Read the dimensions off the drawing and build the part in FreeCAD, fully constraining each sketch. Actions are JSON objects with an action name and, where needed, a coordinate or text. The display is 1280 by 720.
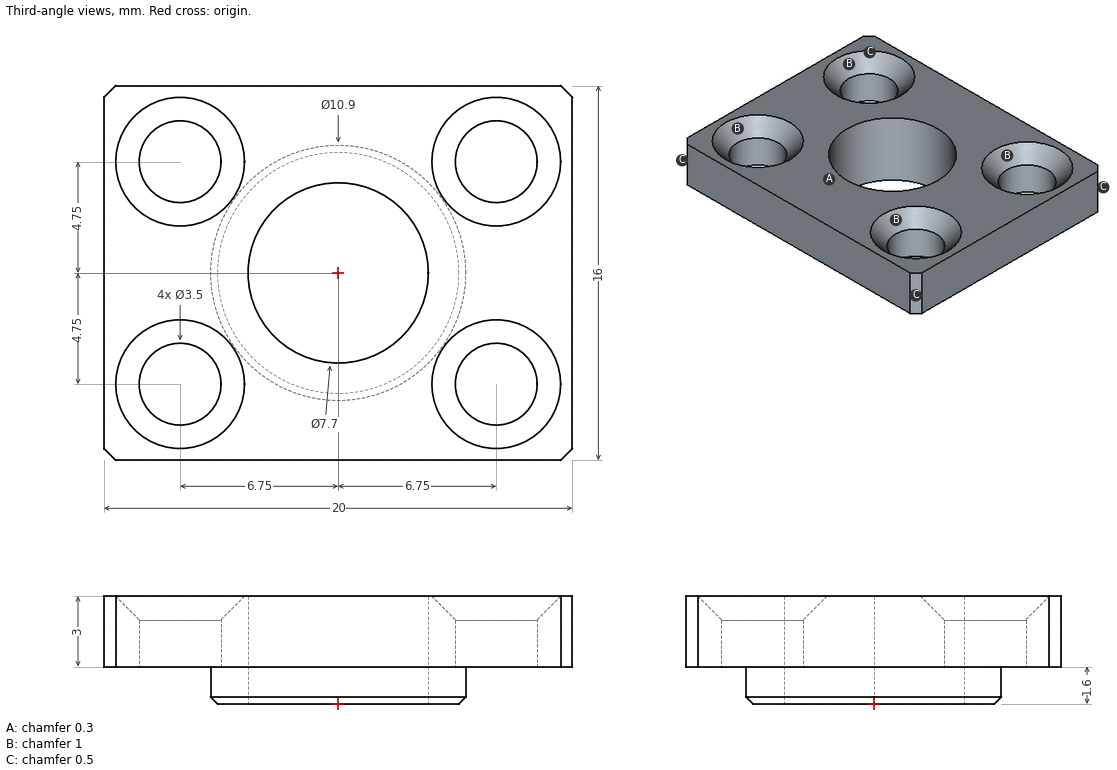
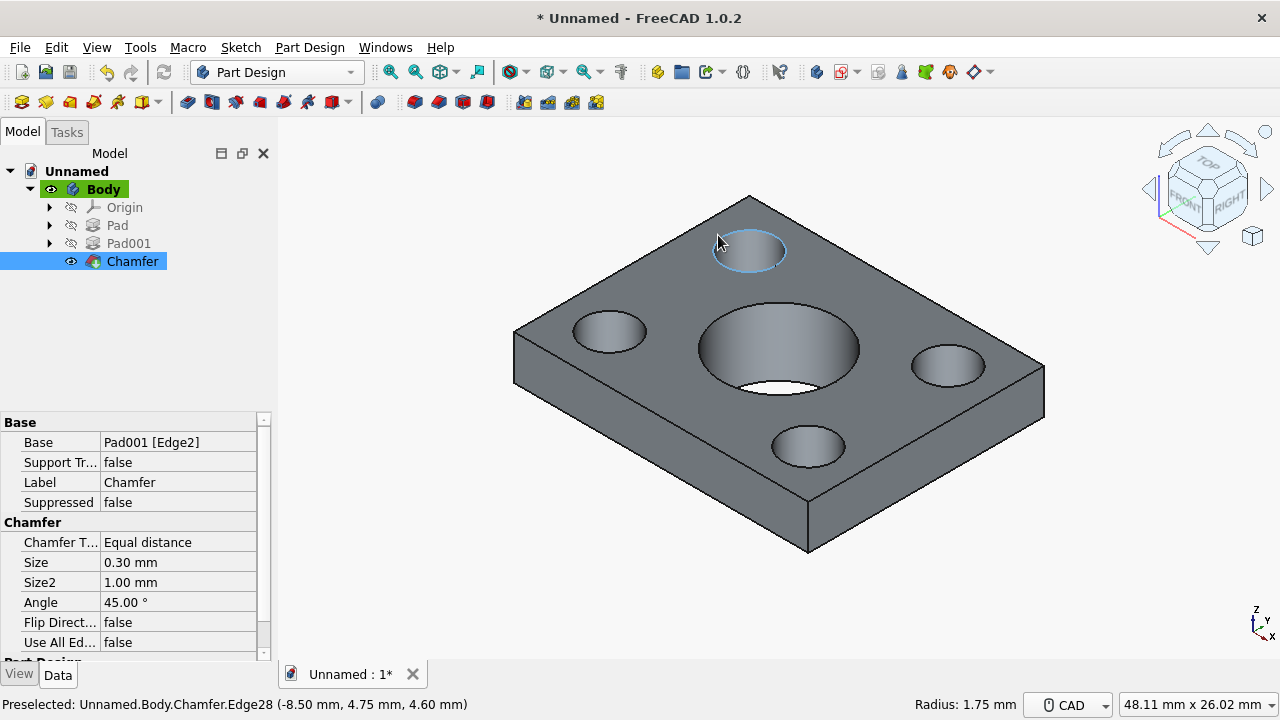
{"action": "left_click", "coordinate": [584, 316], "text": "ctrl"}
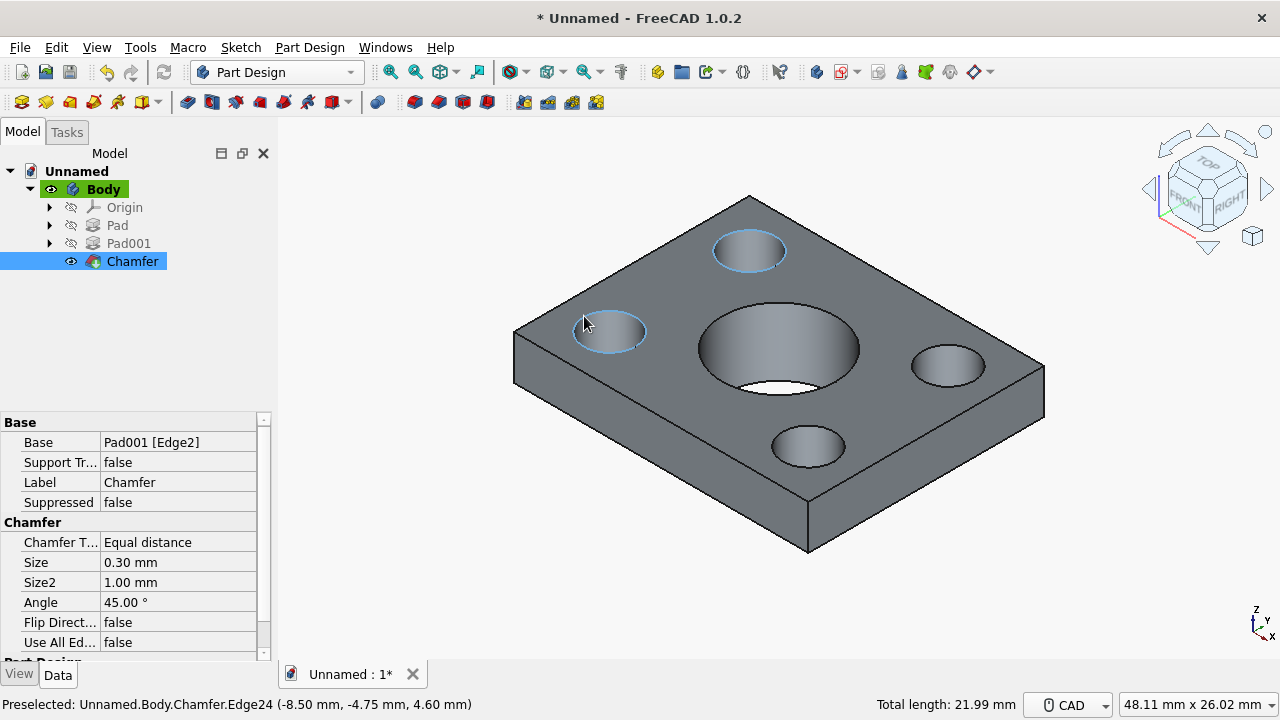
{"action": "left_click", "coordinate": [783, 431], "text": "ctrl"}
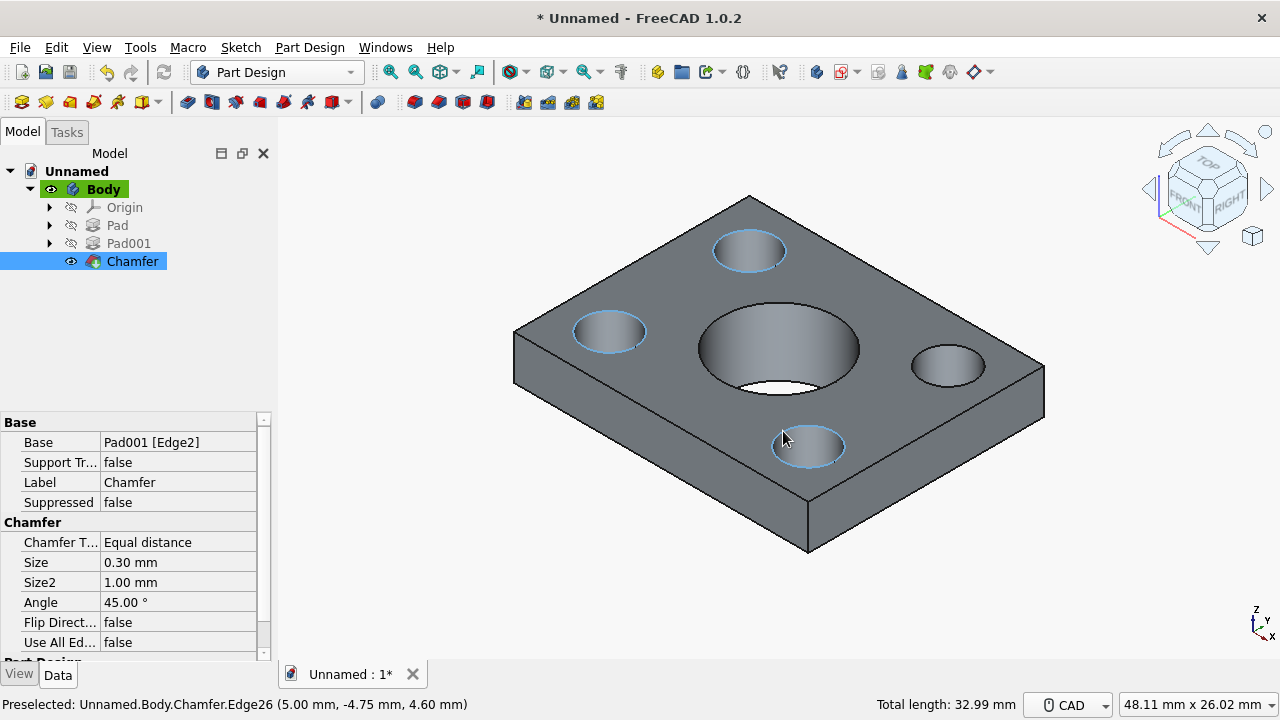
{"action": "left_click", "coordinate": [923, 350], "text": "ctrl"}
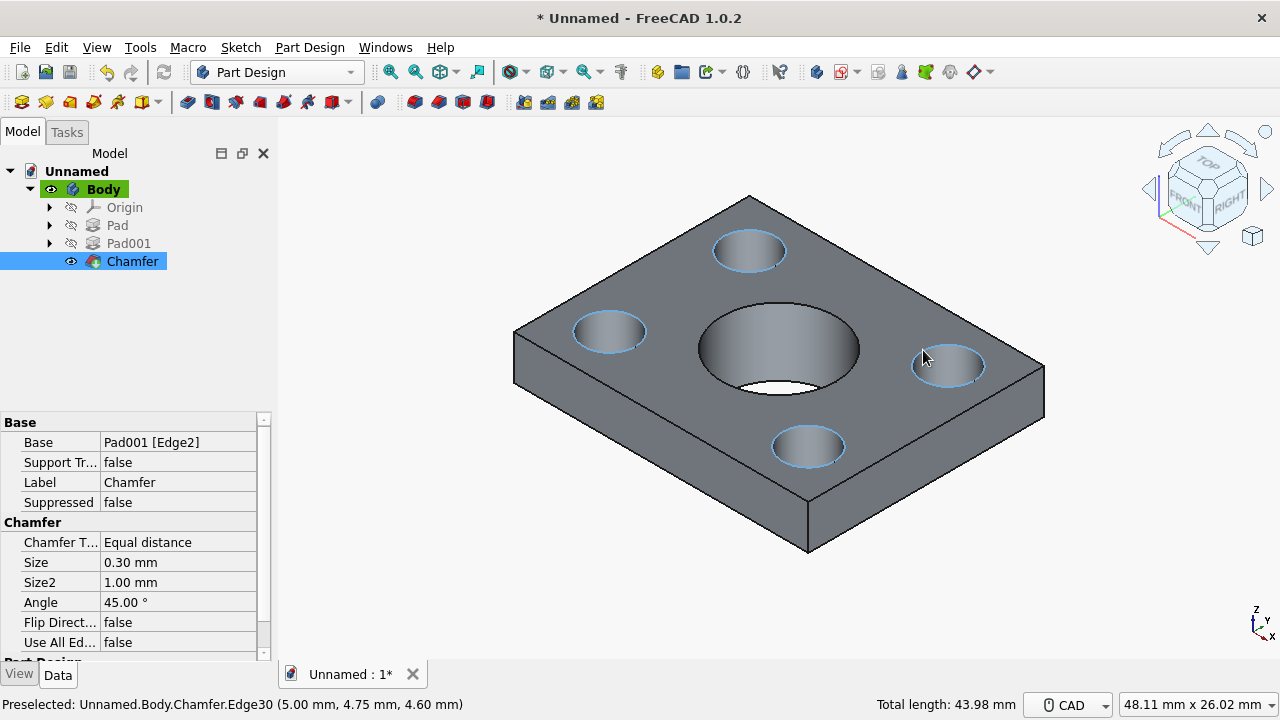
{"action": "left_click", "coordinate": [440, 102]}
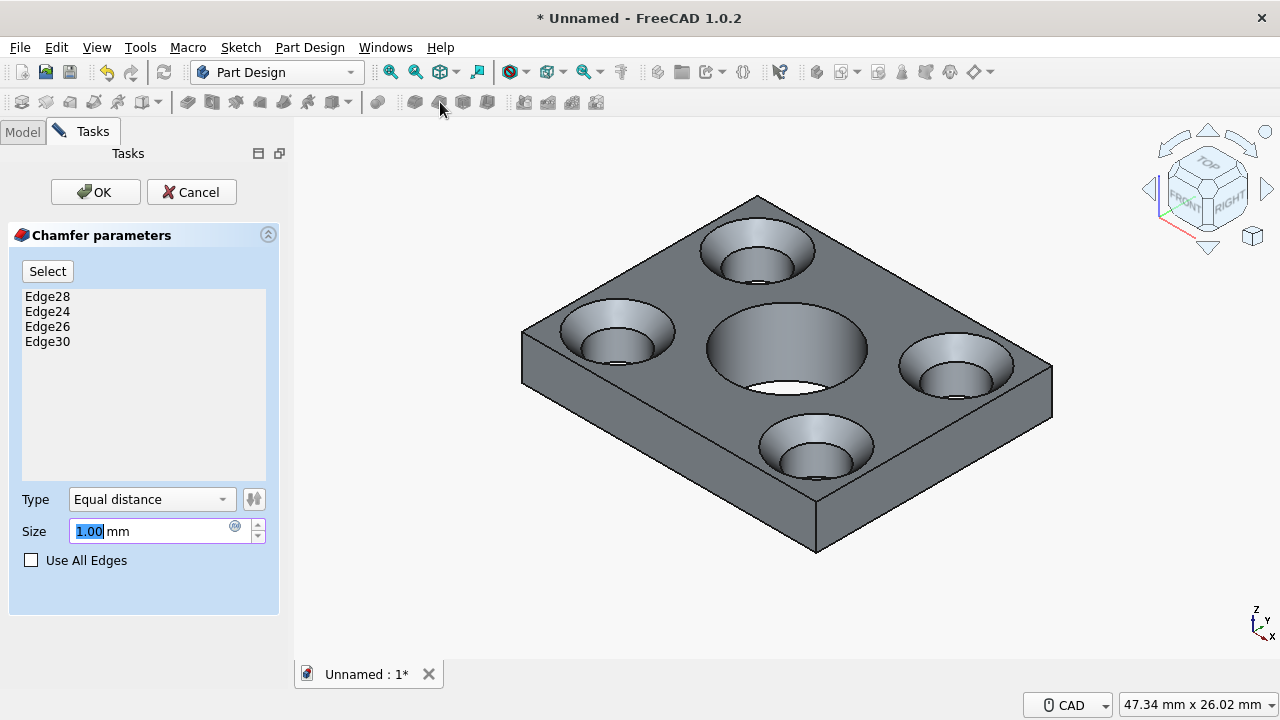
{"action": "type", "text": "1"}
{"action": "key", "text": "Tab"}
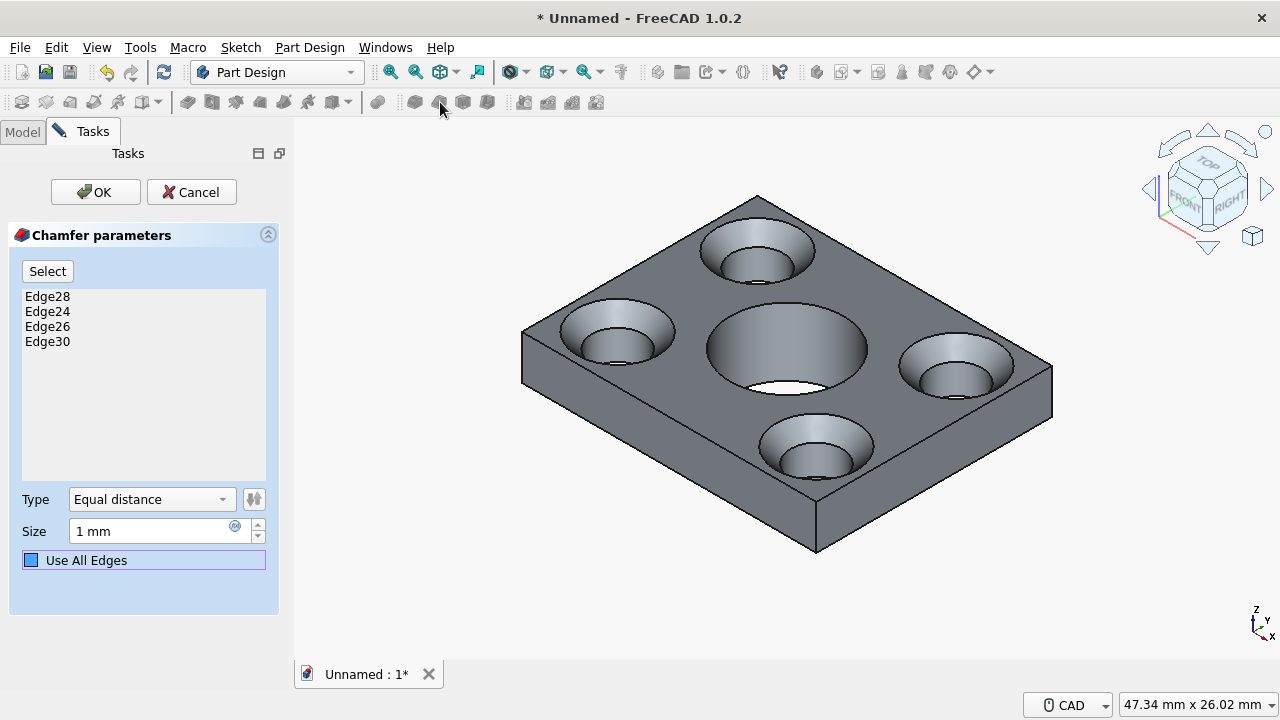
{"action": "left_click", "coordinate": [96, 192]}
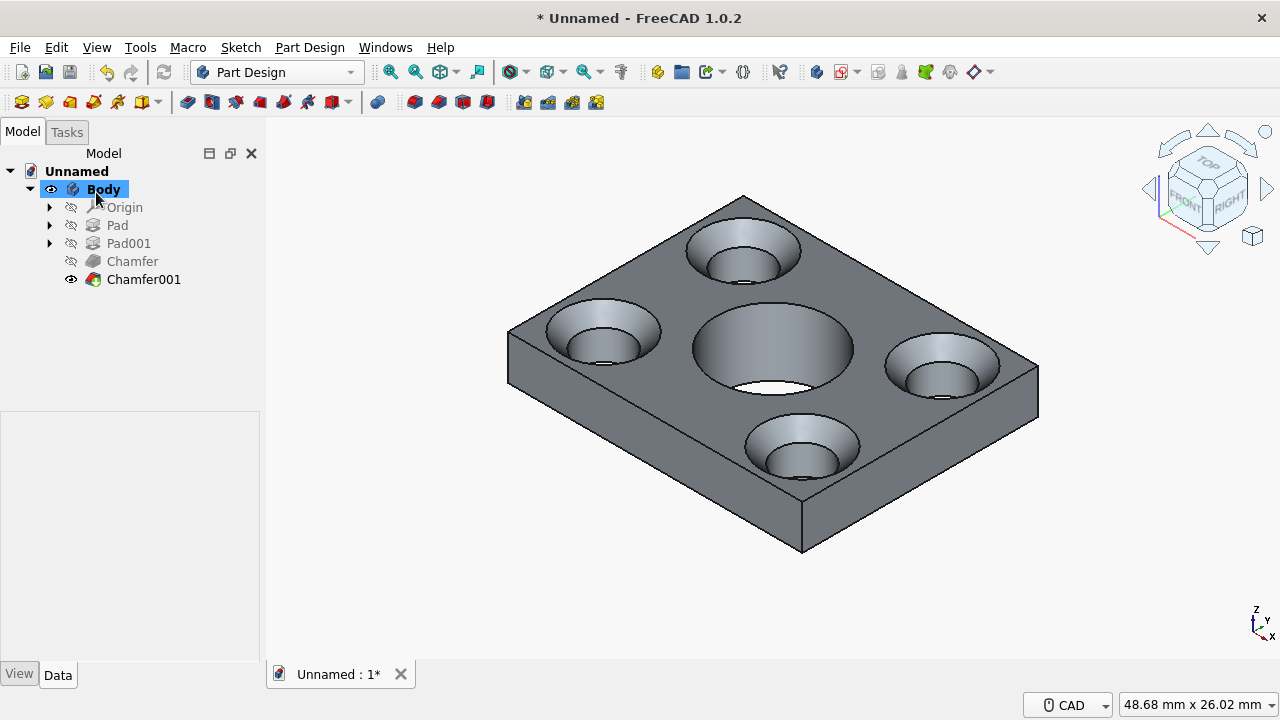
{"action": "left_click", "coordinate": [802, 526]}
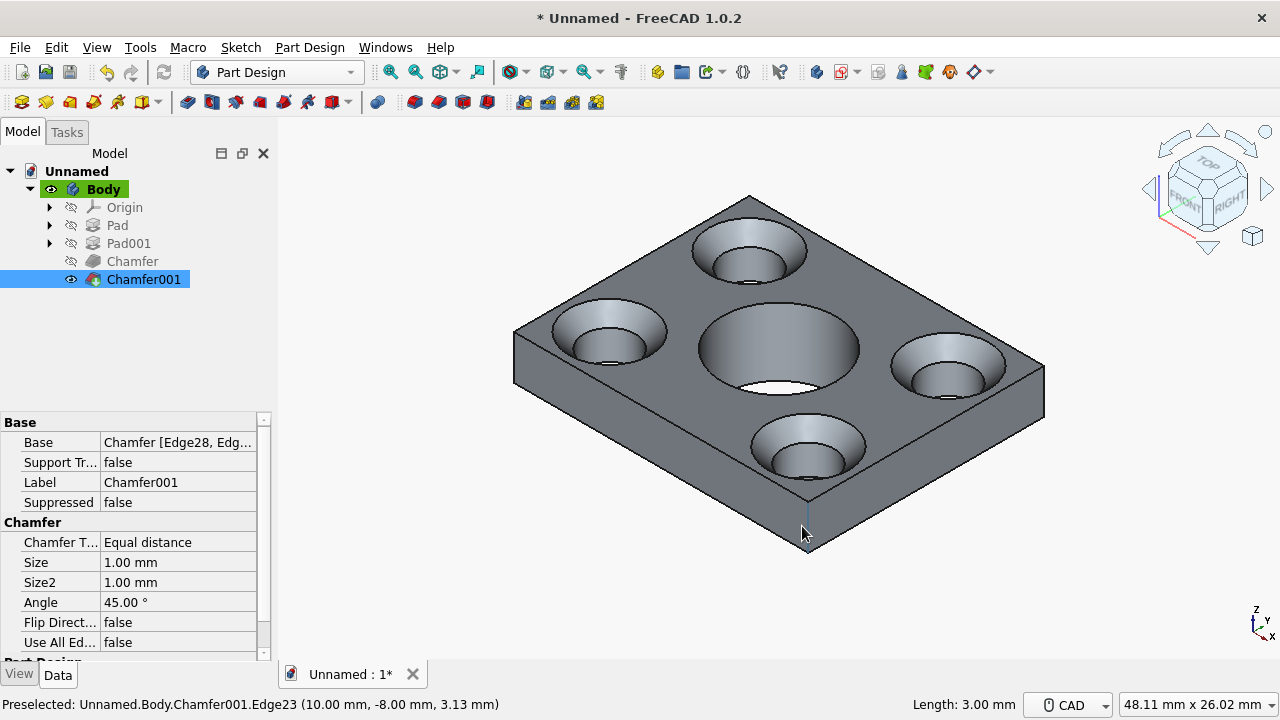
{"action": "key", "text": "2"}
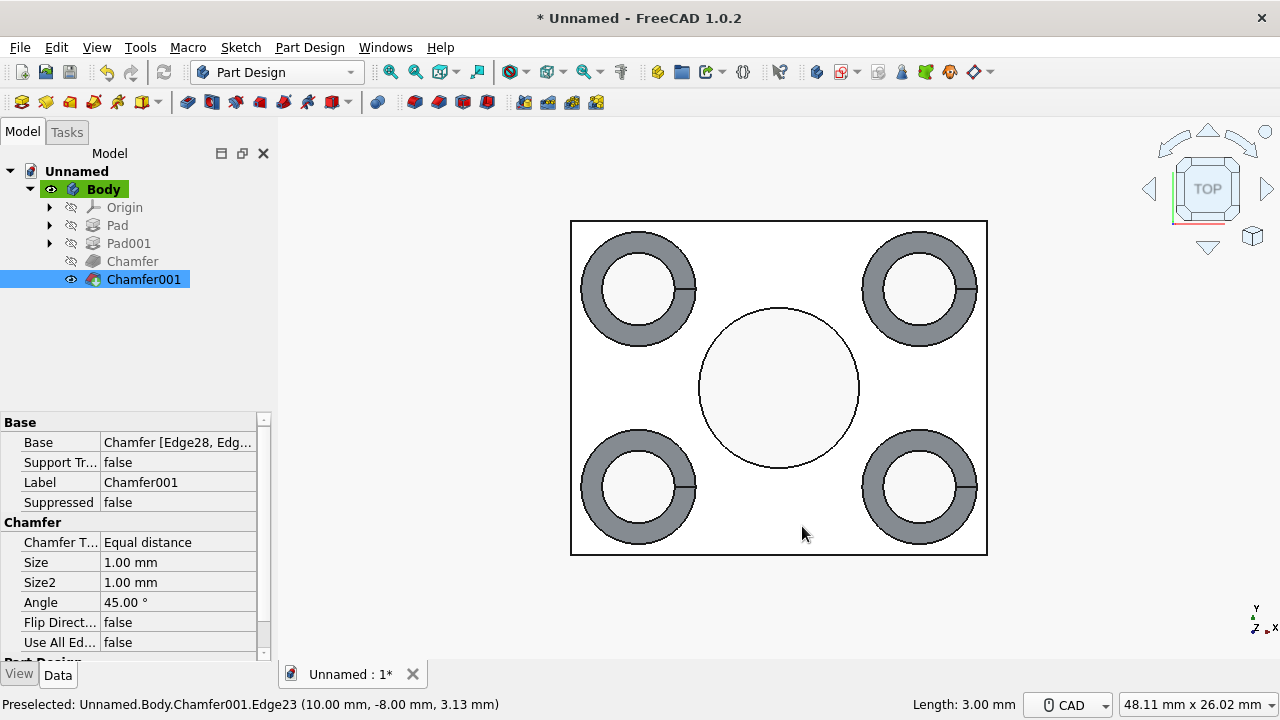
{"action": "key", "text": "0"}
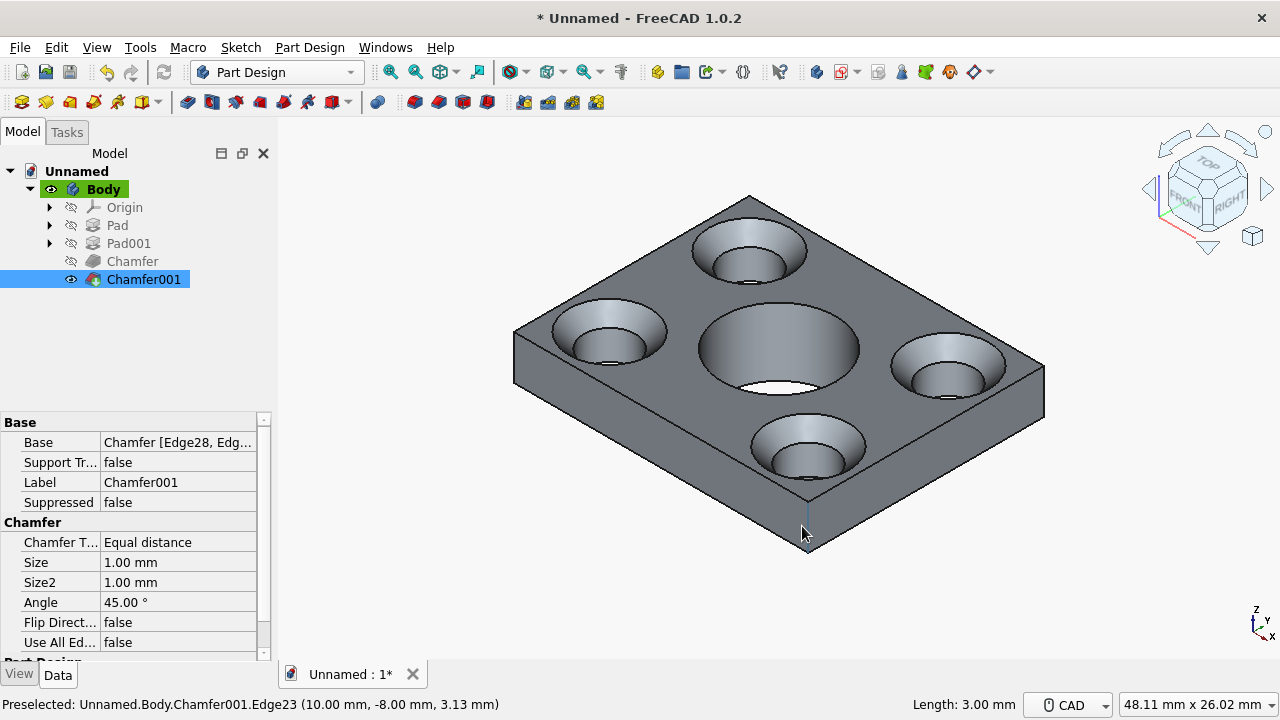
{"action": "key", "text": "1"}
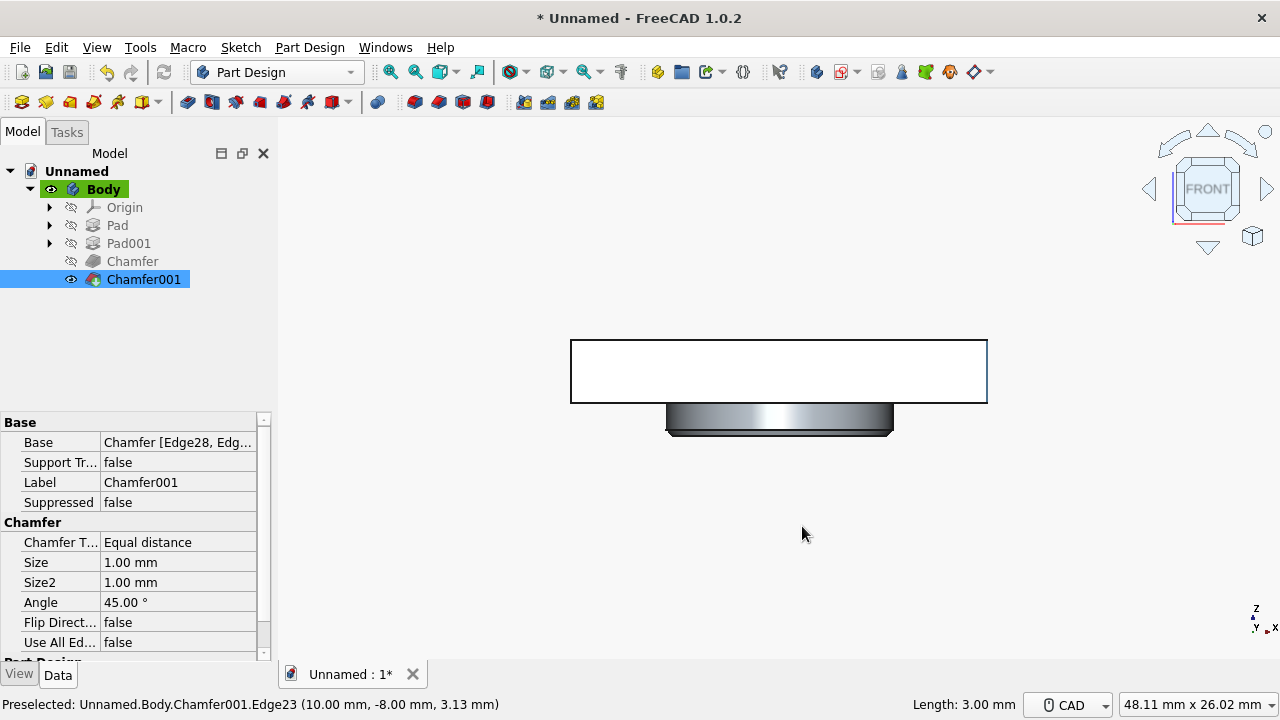
{"action": "left_click", "coordinate": [392, 72]}